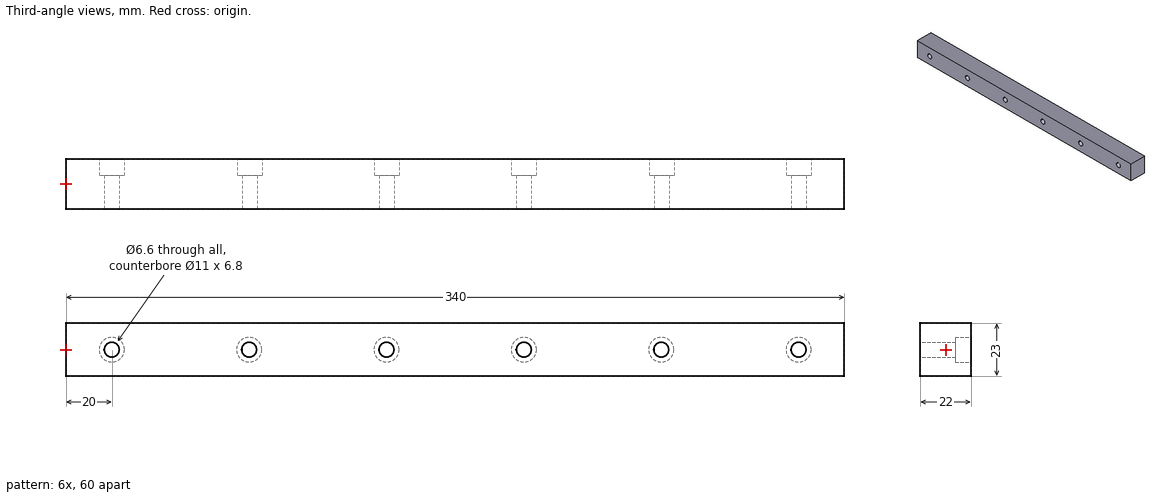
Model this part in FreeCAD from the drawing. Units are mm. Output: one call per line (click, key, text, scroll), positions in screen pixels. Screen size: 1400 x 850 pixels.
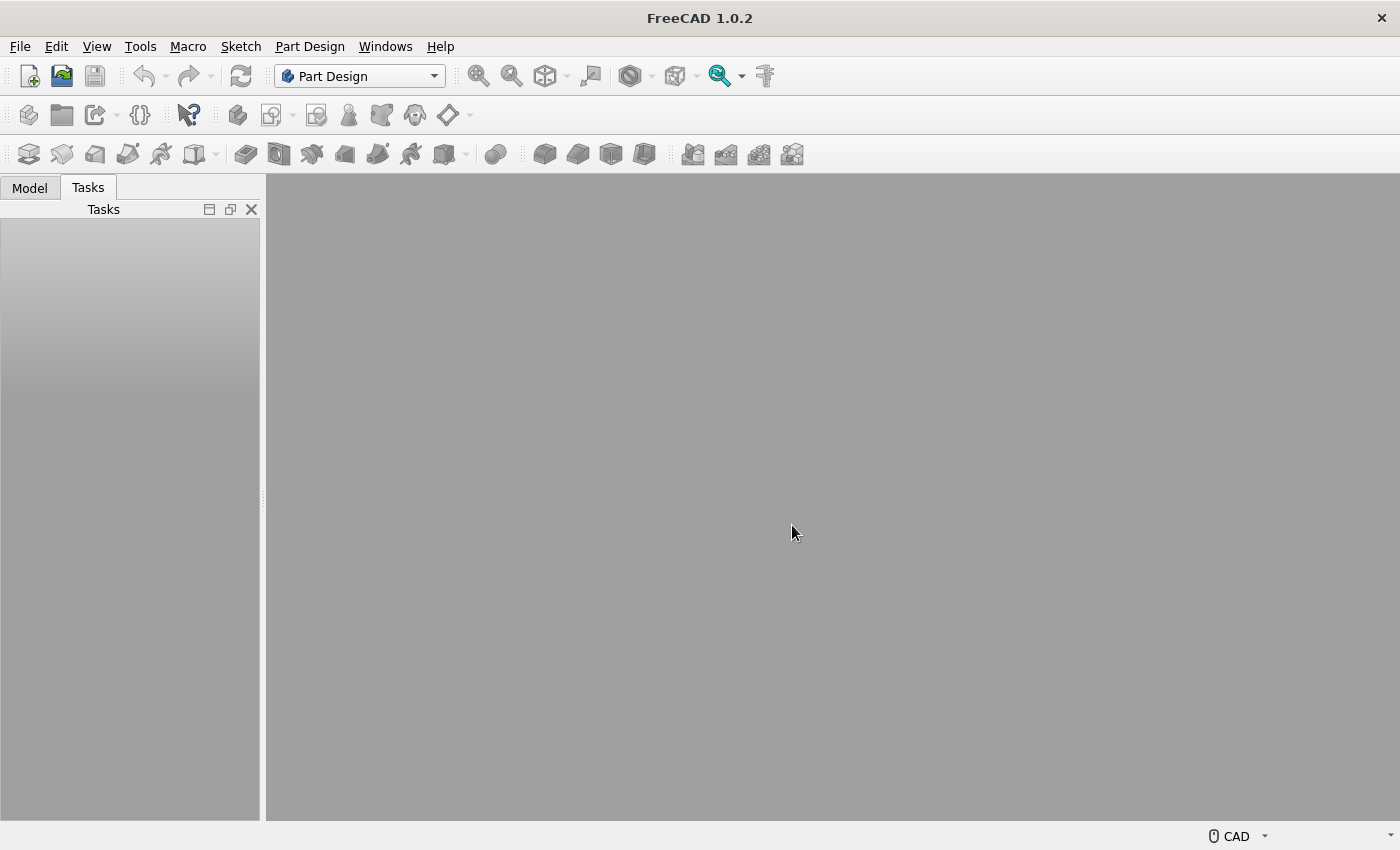
key(ctrl+n)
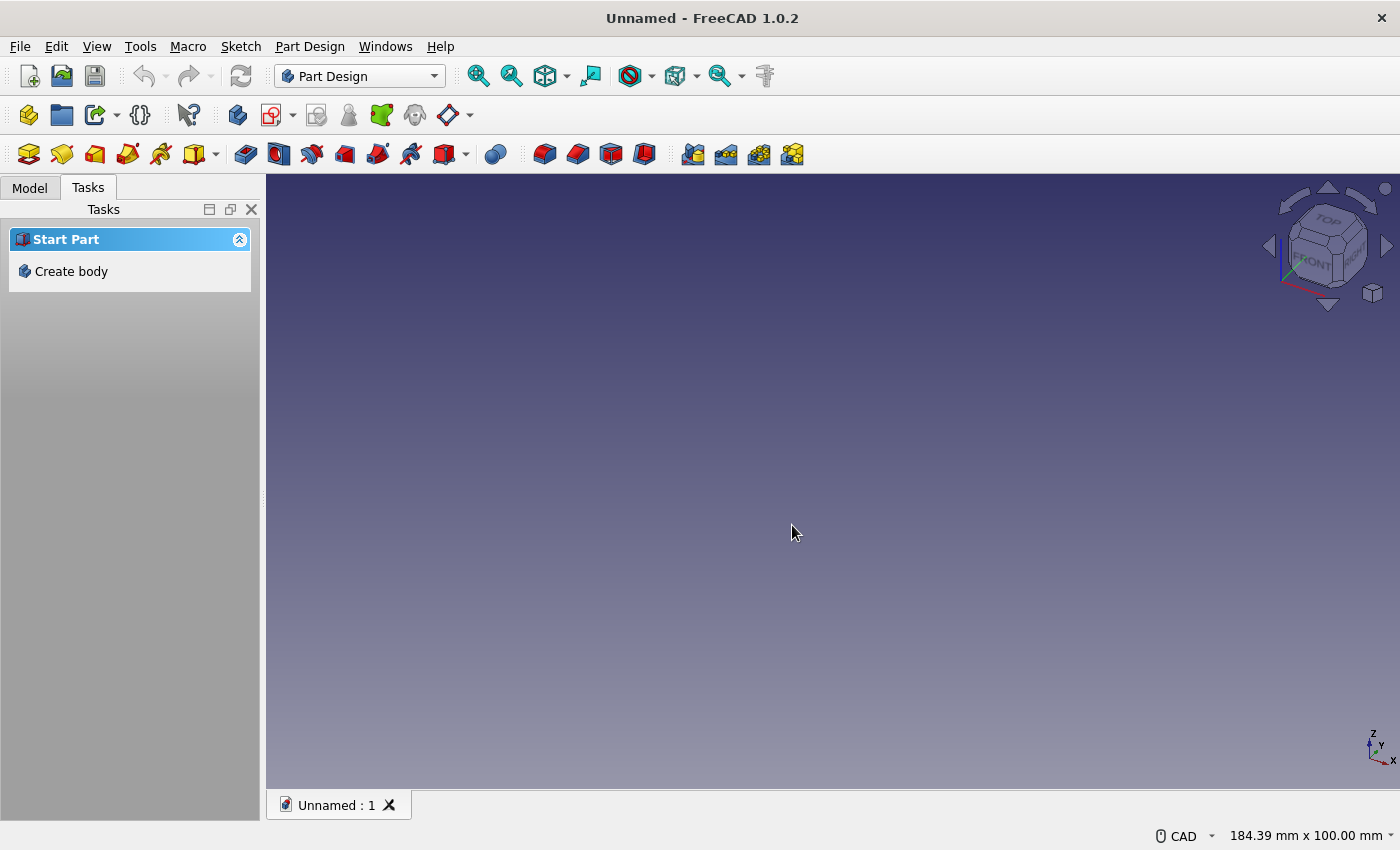
click(270, 116)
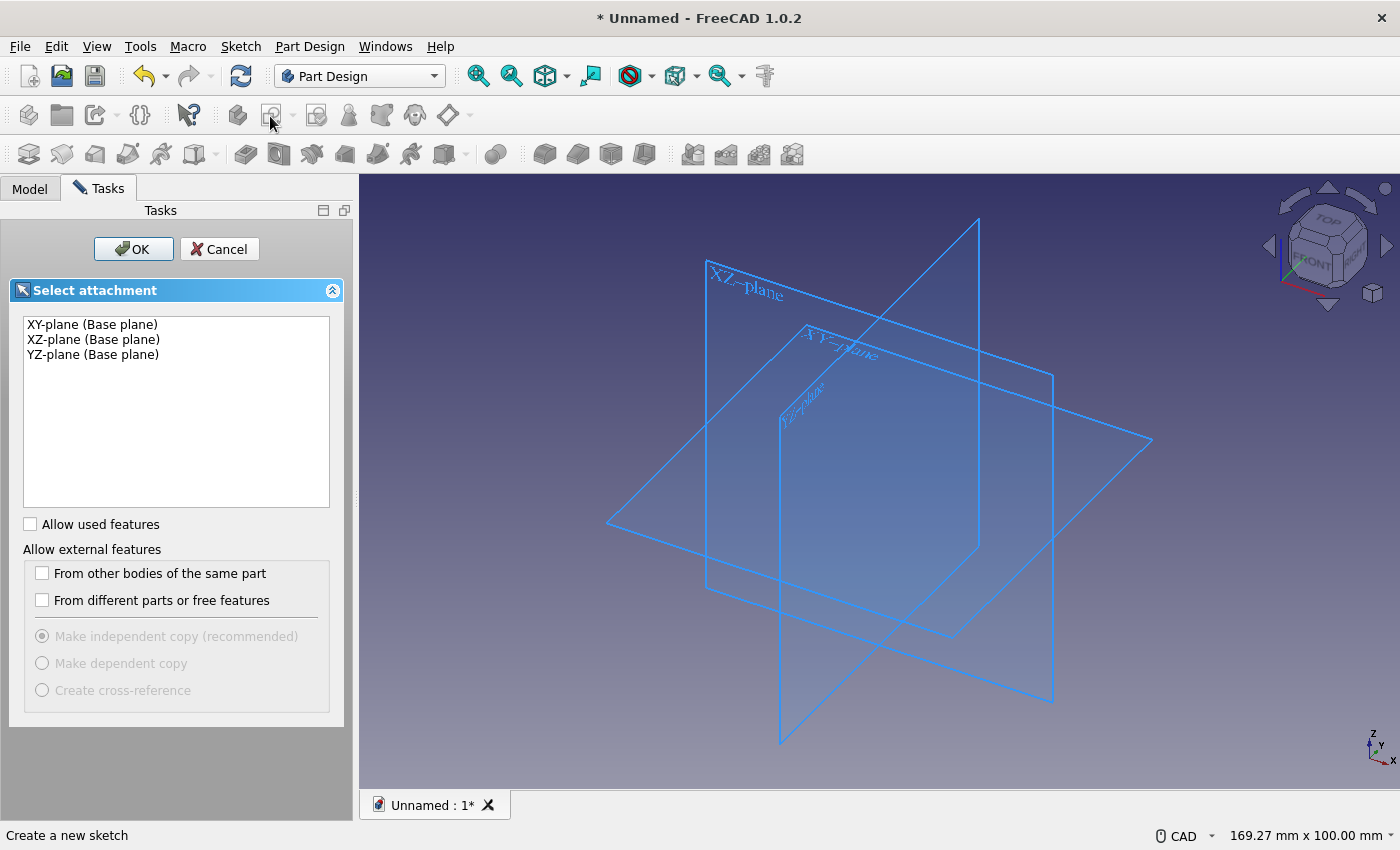
click(84, 354)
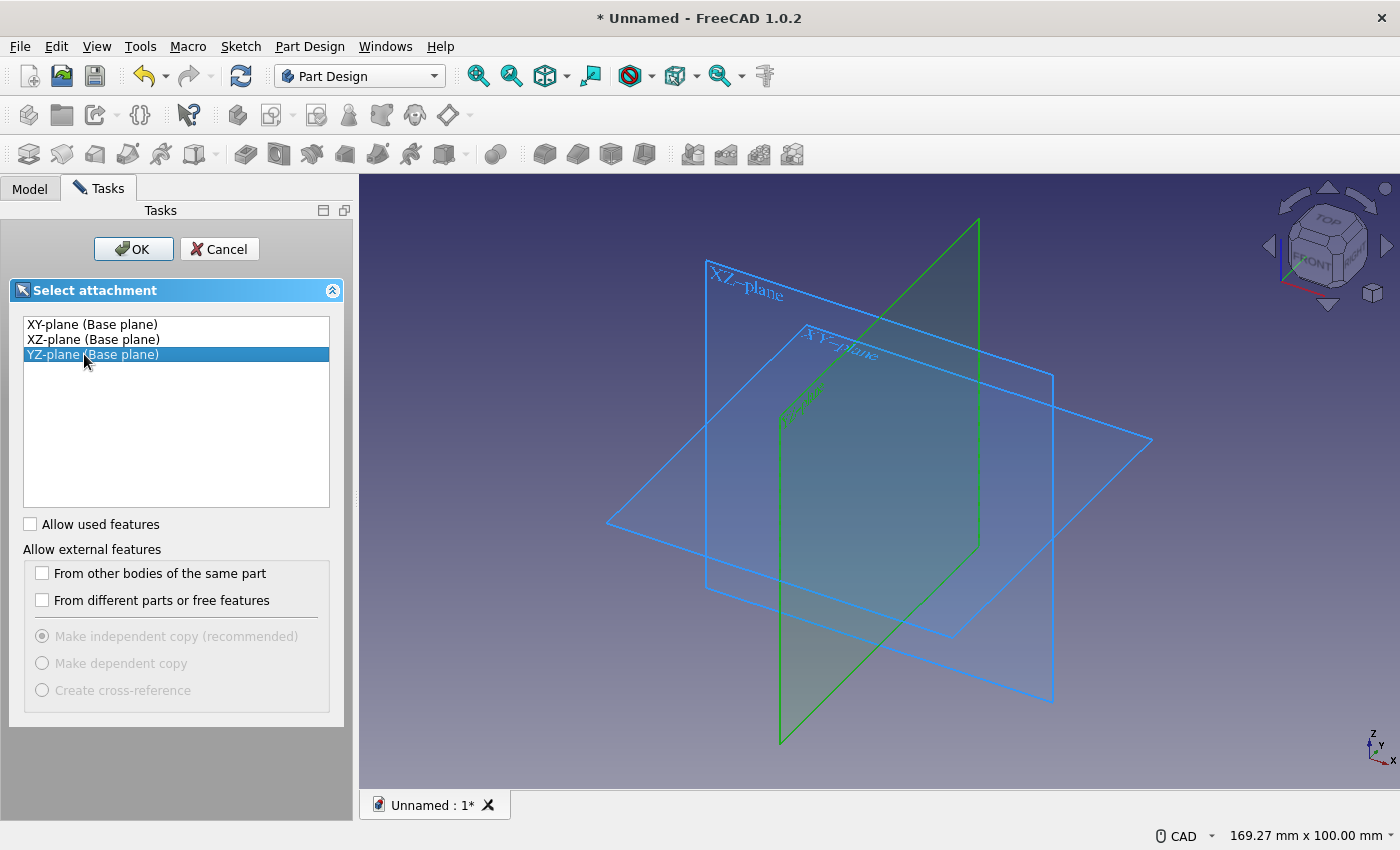
click(134, 249)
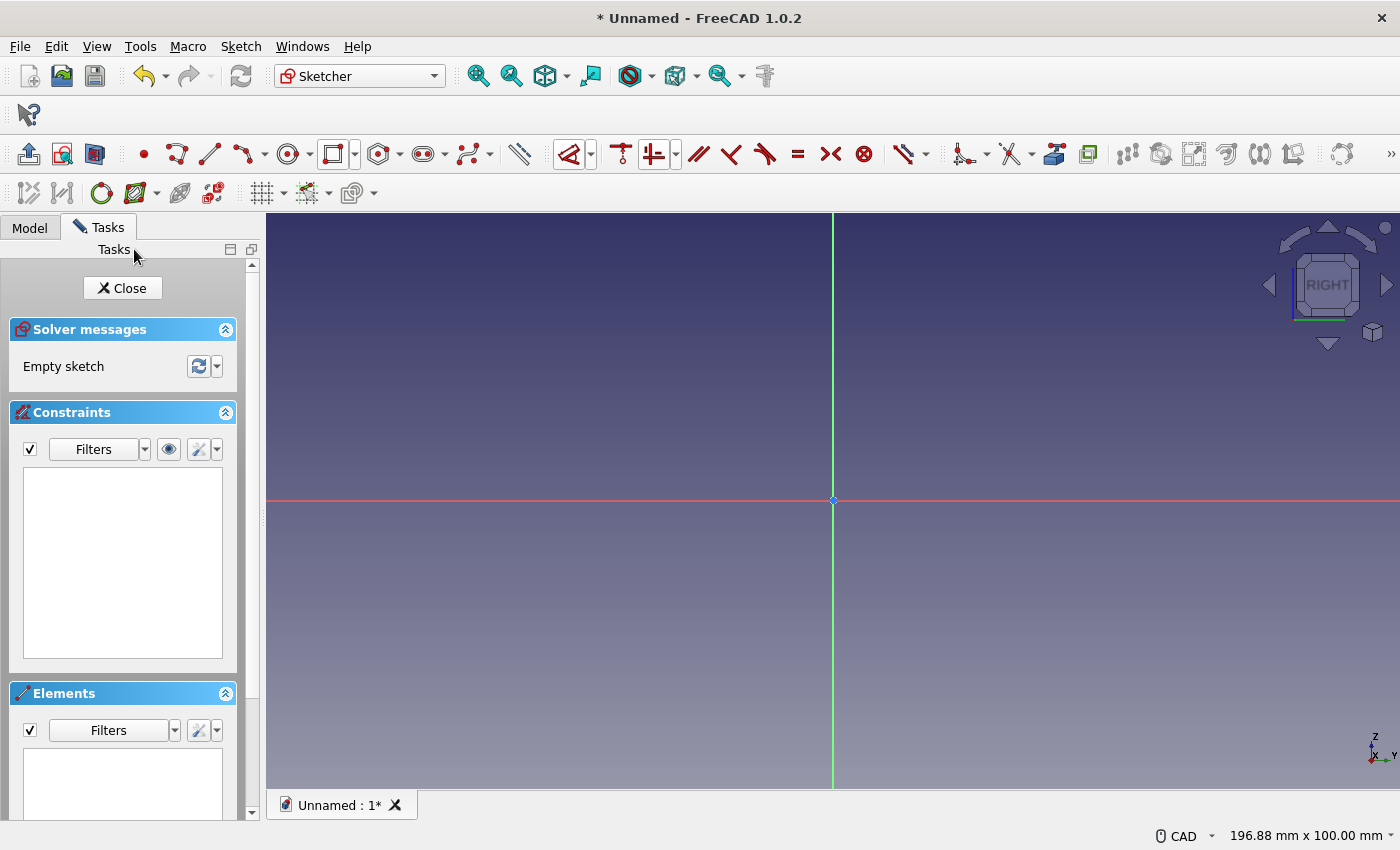
scroll(873, 501, up, 5)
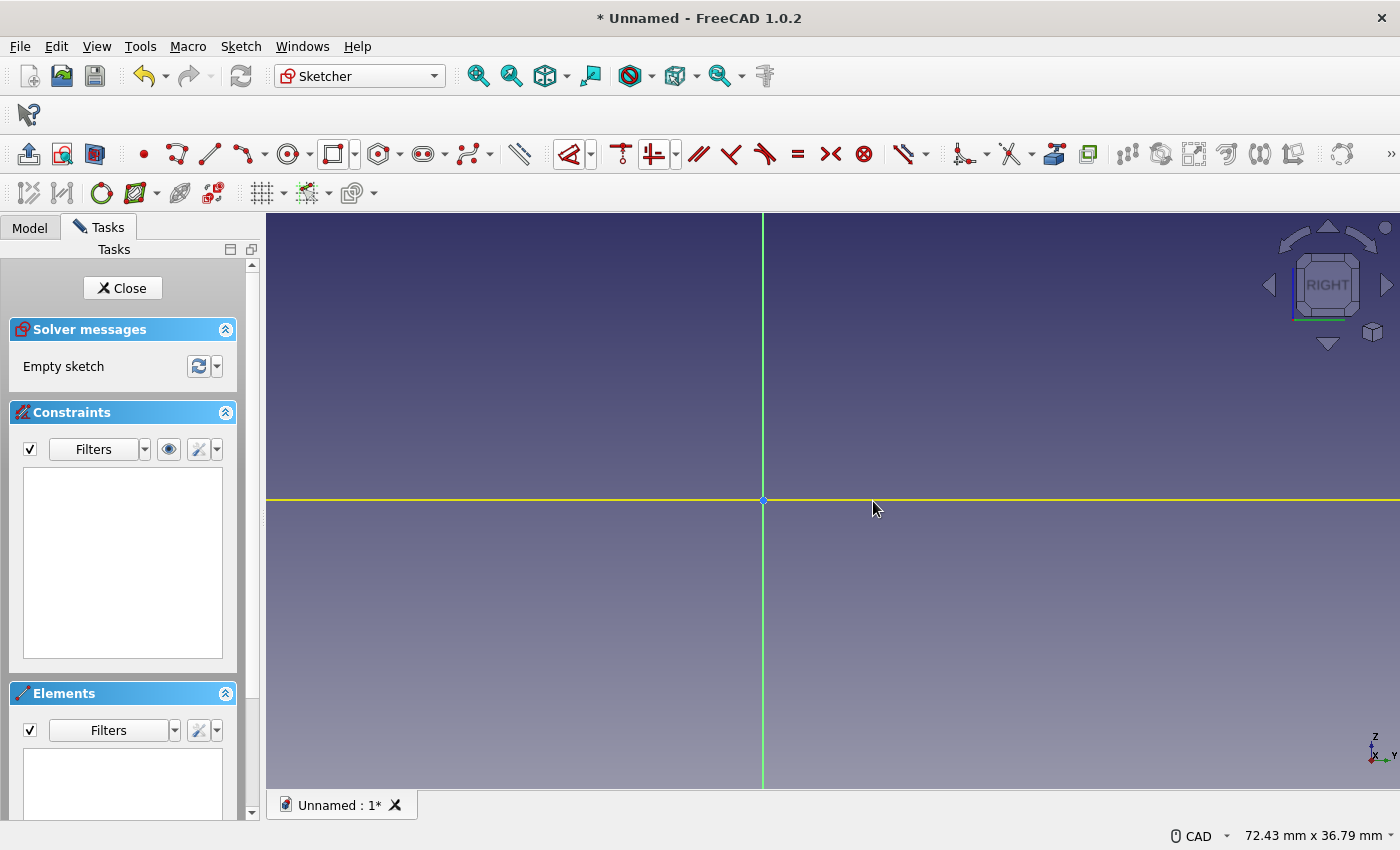
click(354, 154)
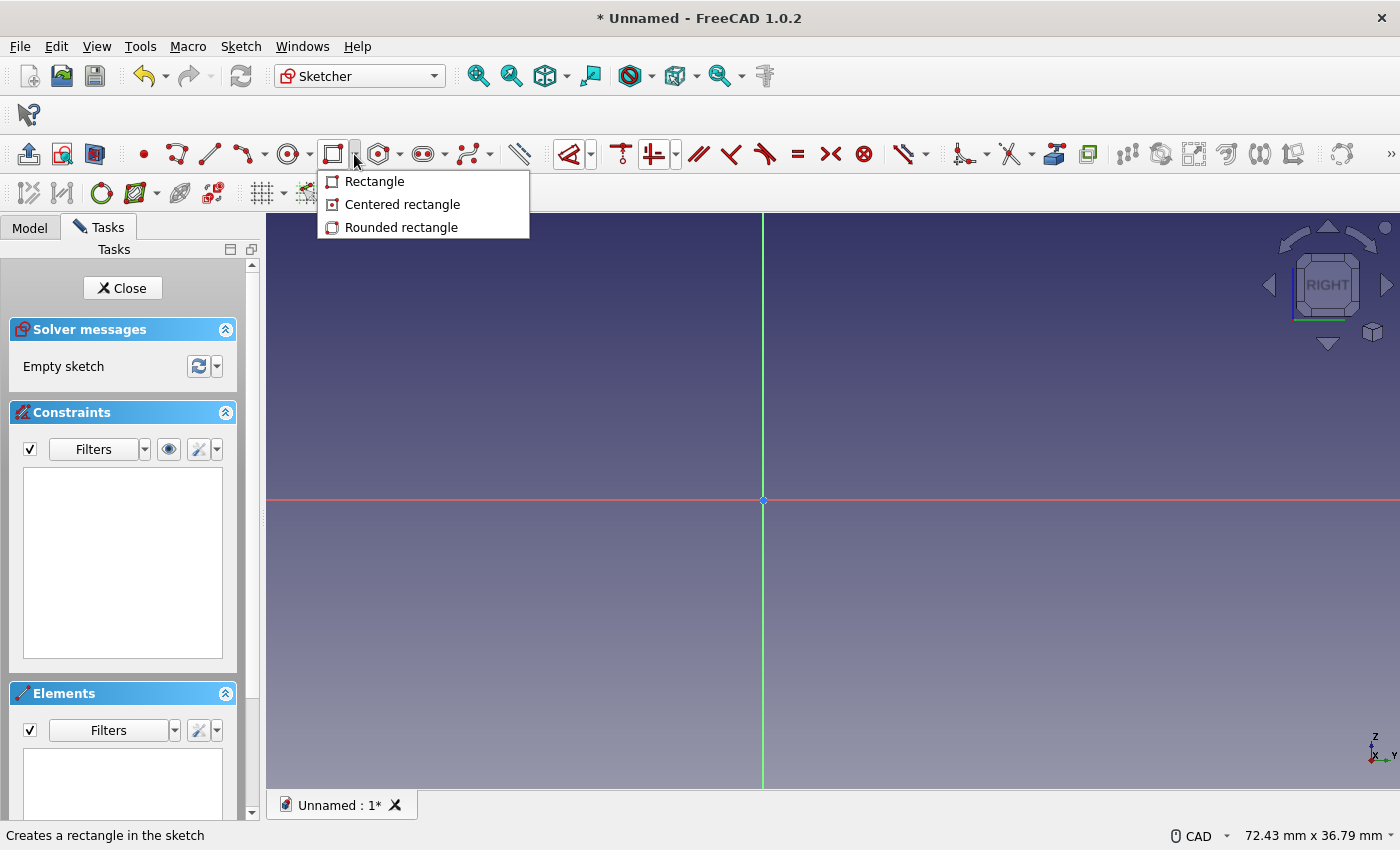
click(424, 204)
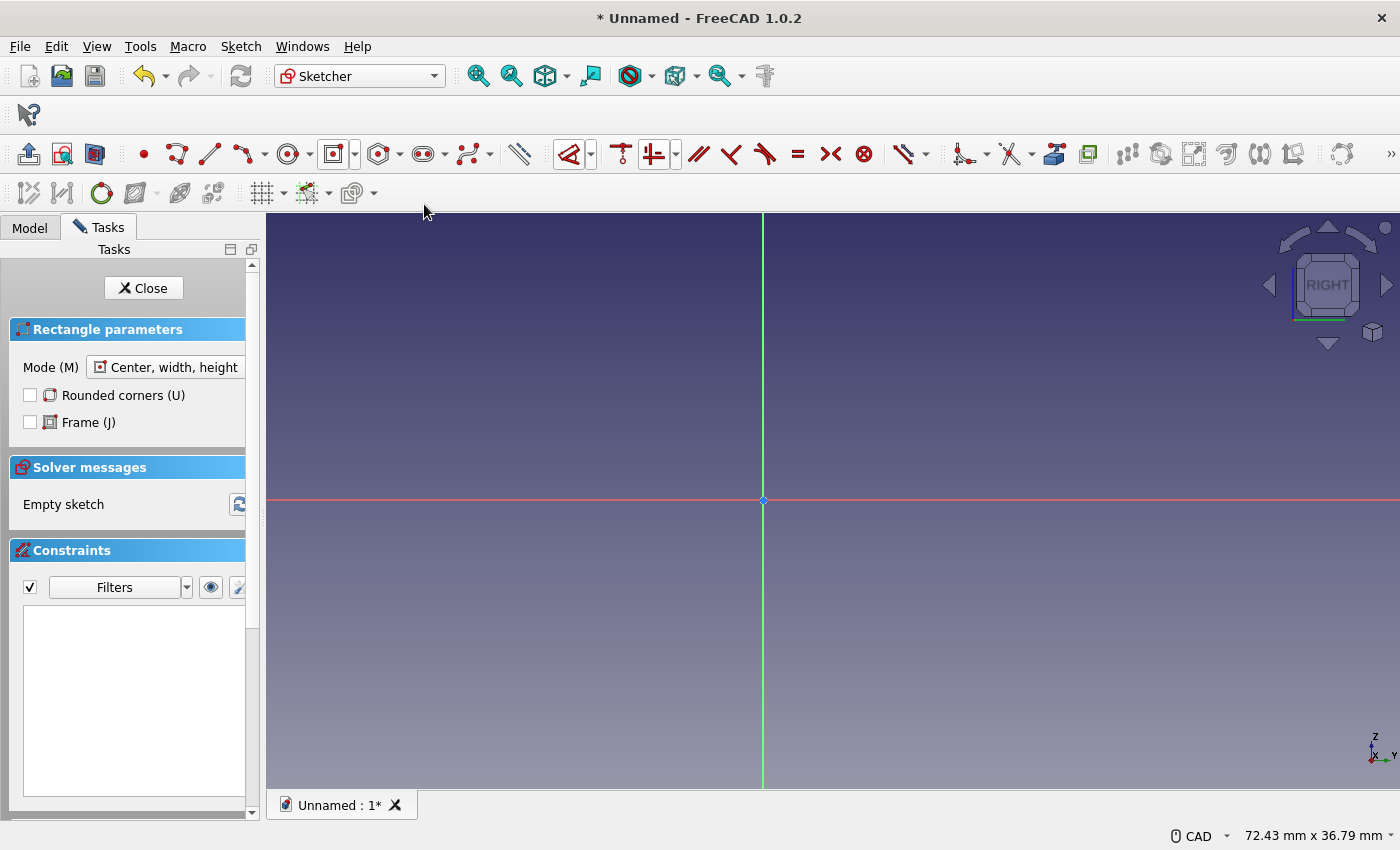
click(763, 500)
click(936, 320)
key(Escape)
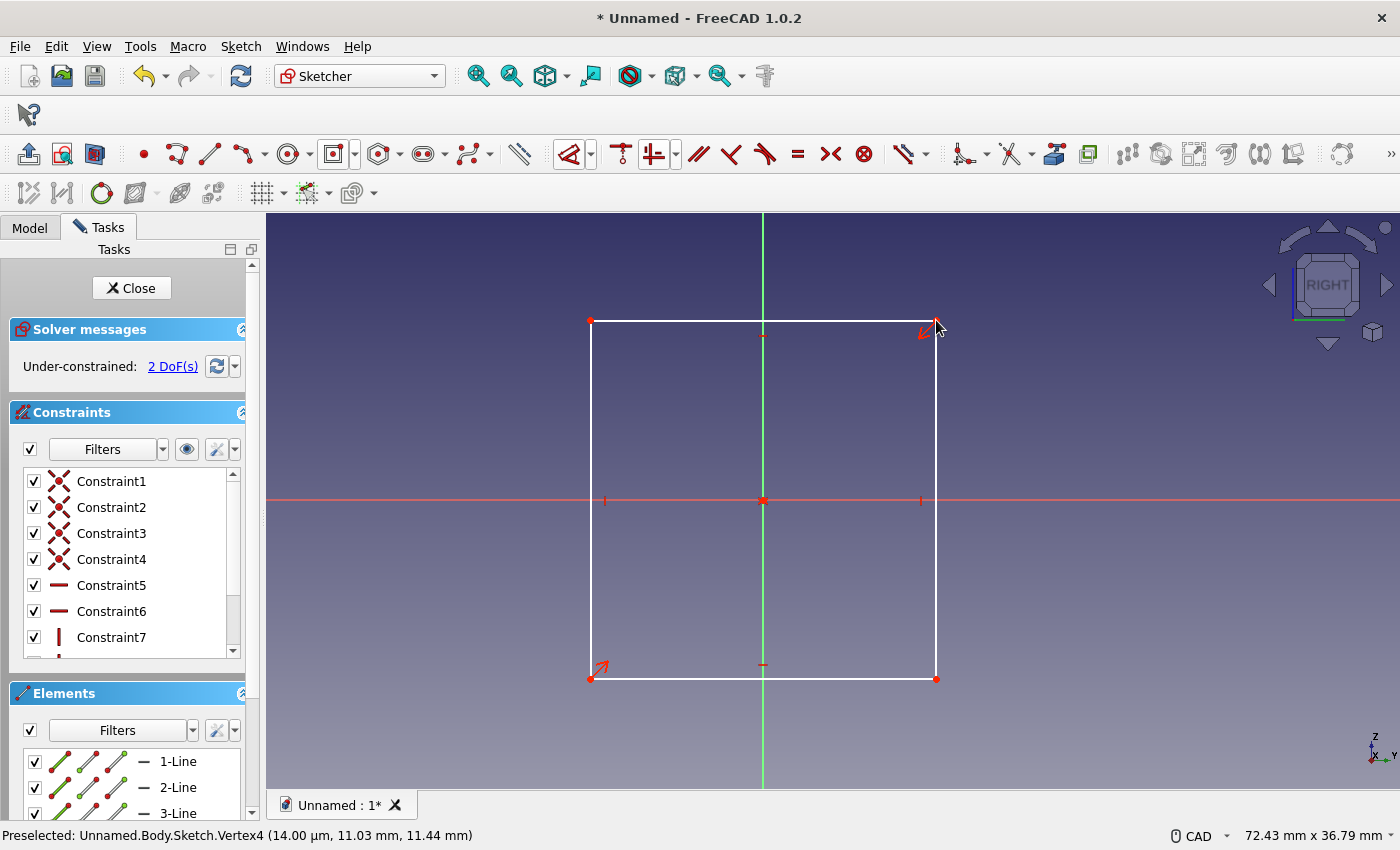
key(d)